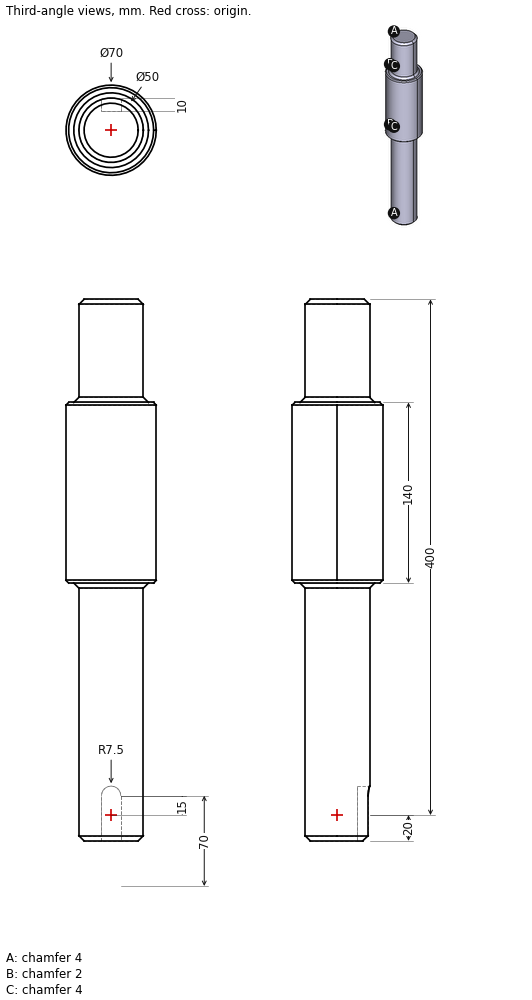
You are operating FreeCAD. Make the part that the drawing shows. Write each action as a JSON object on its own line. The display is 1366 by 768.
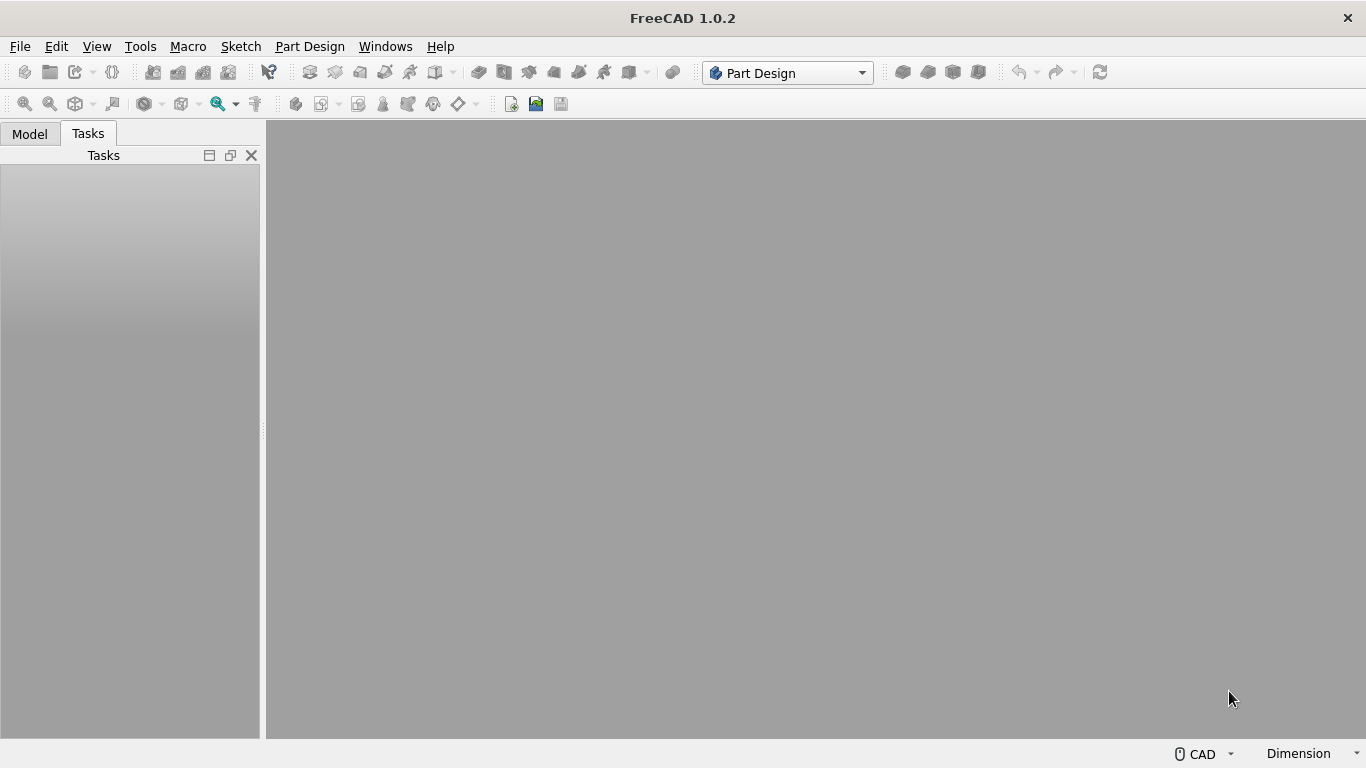
{"action": "left_click", "coordinate": [511, 104]}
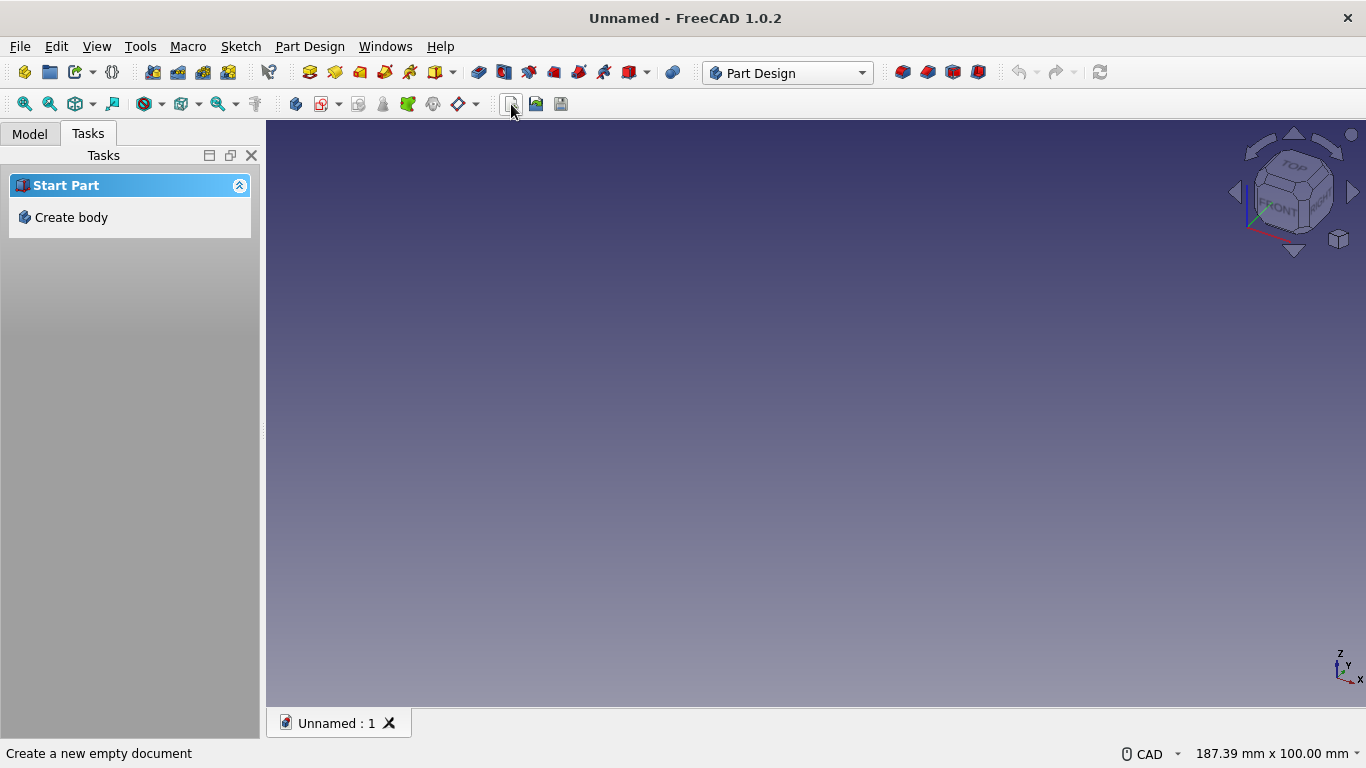
{"action": "left_click", "coordinate": [320, 104]}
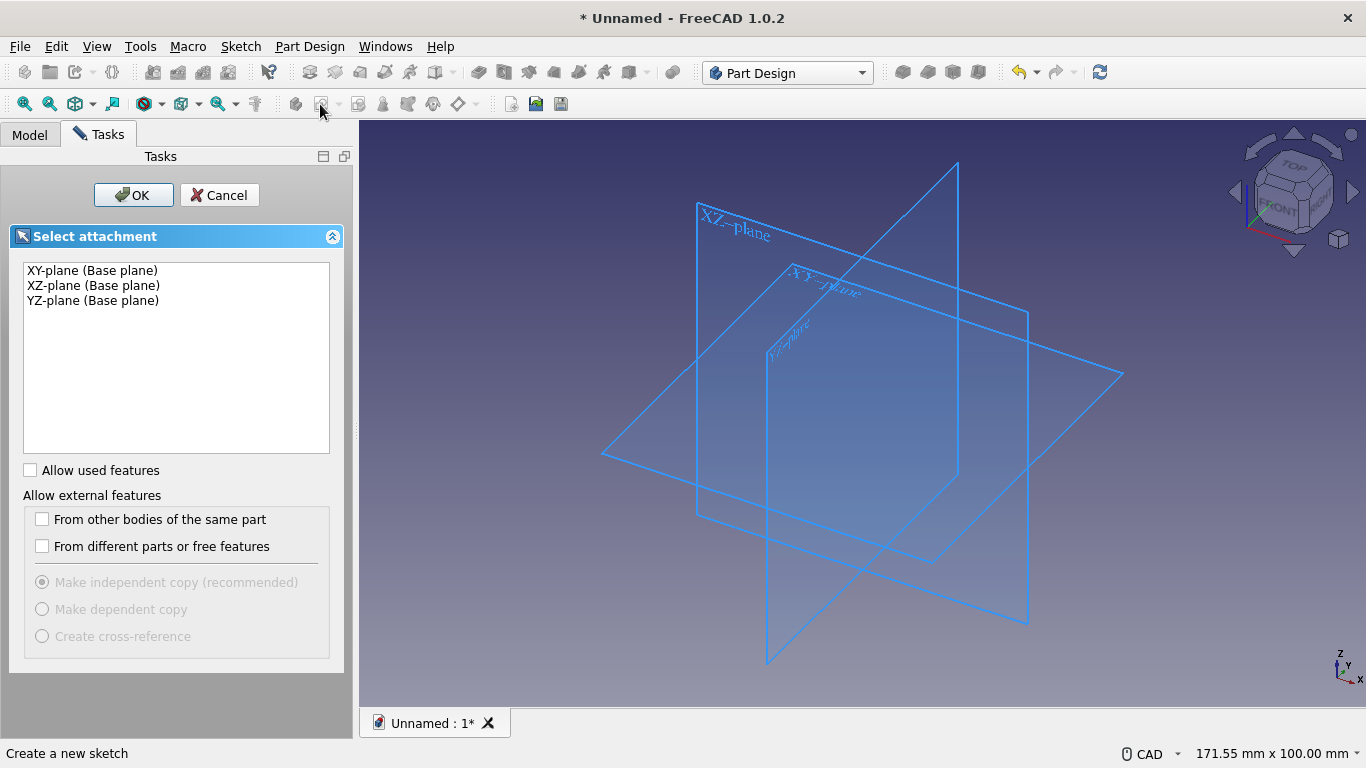
{"action": "left_click", "coordinate": [84, 270]}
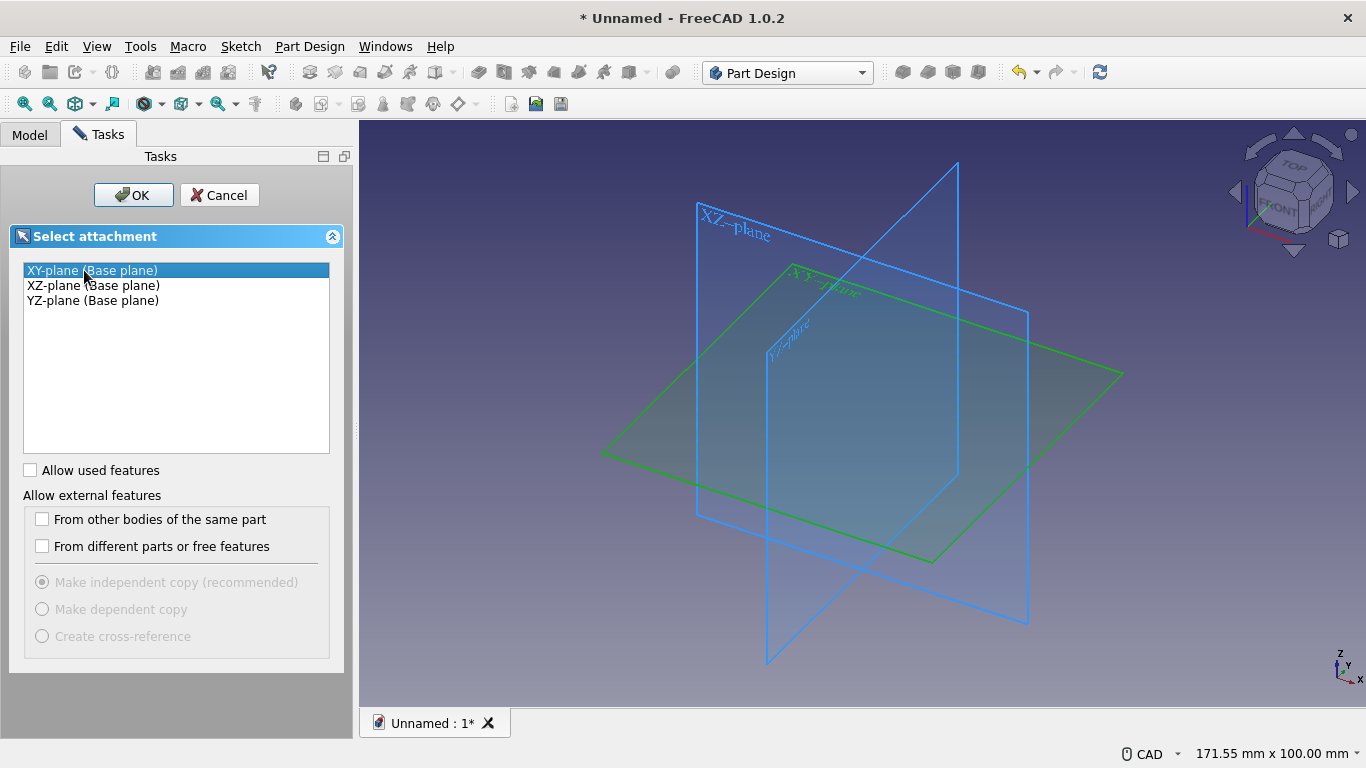
{"action": "left_click", "coordinate": [134, 195]}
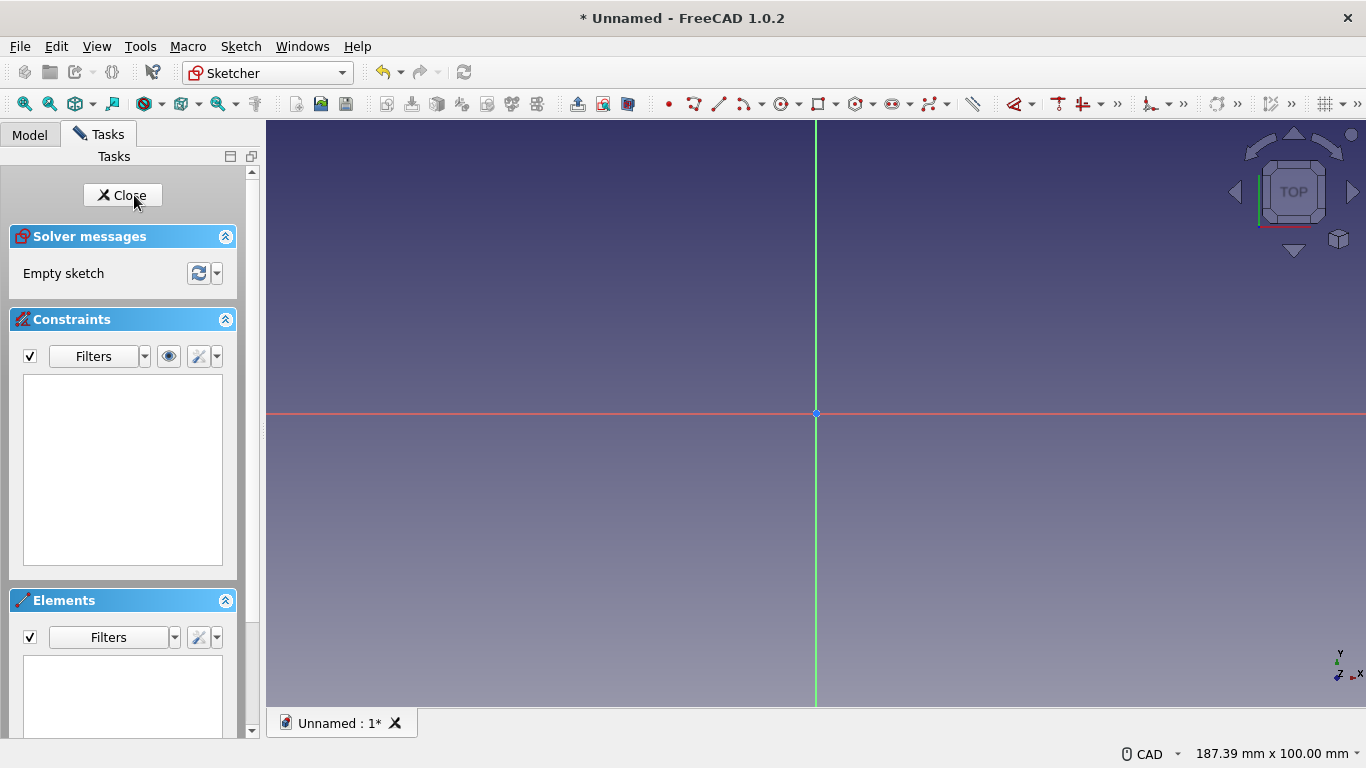
{"action": "left_click", "coordinate": [780, 104]}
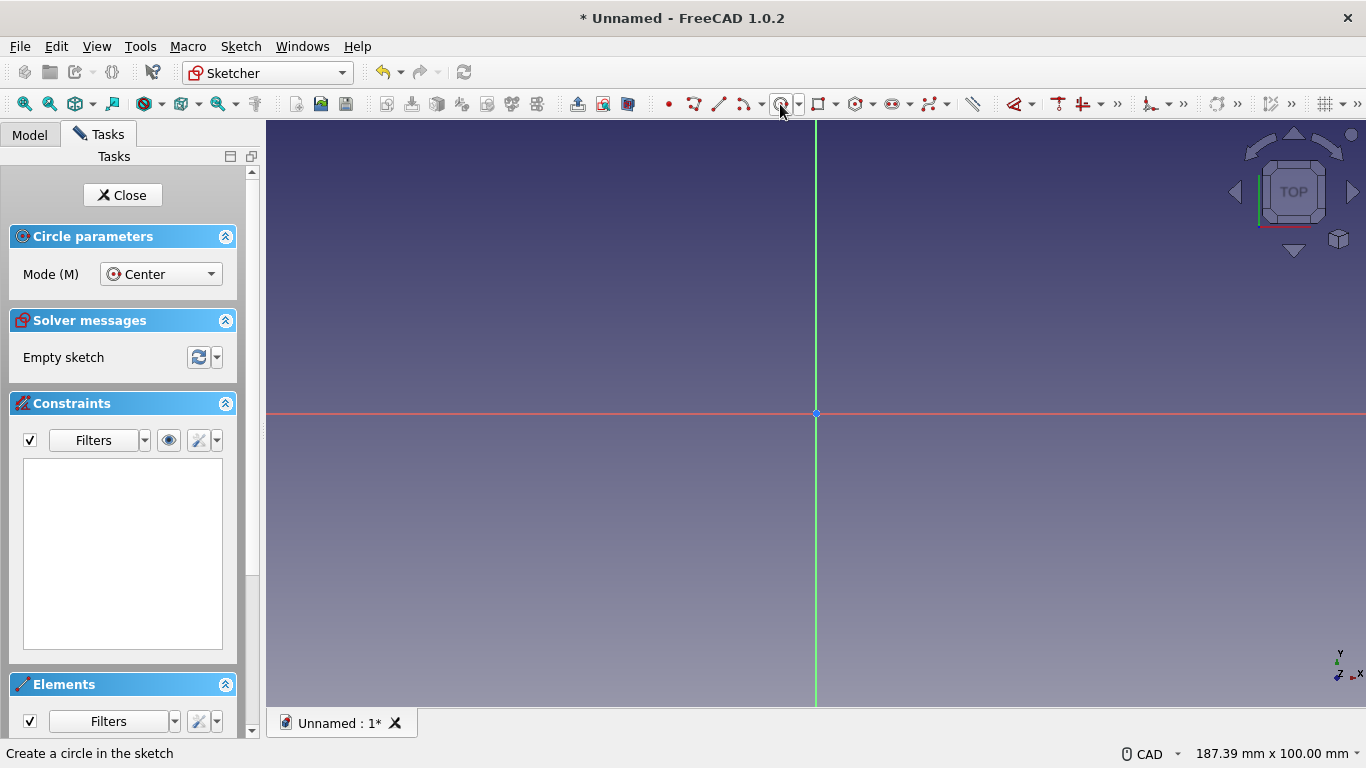
{"action": "left_click", "coordinate": [816, 414]}
{"action": "left_click", "coordinate": [920, 310]}
{"action": "key", "text": "Escape"}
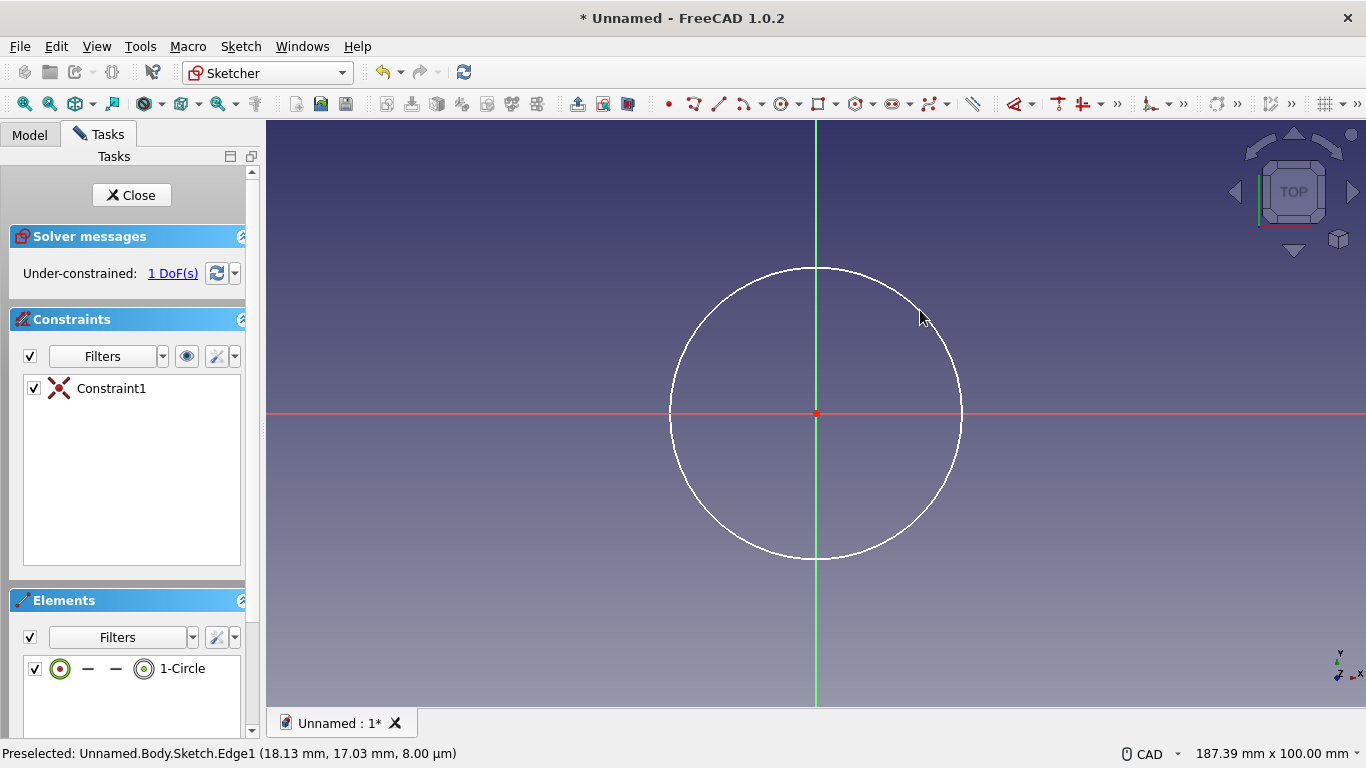
{"action": "left_click", "coordinate": [1014, 104]}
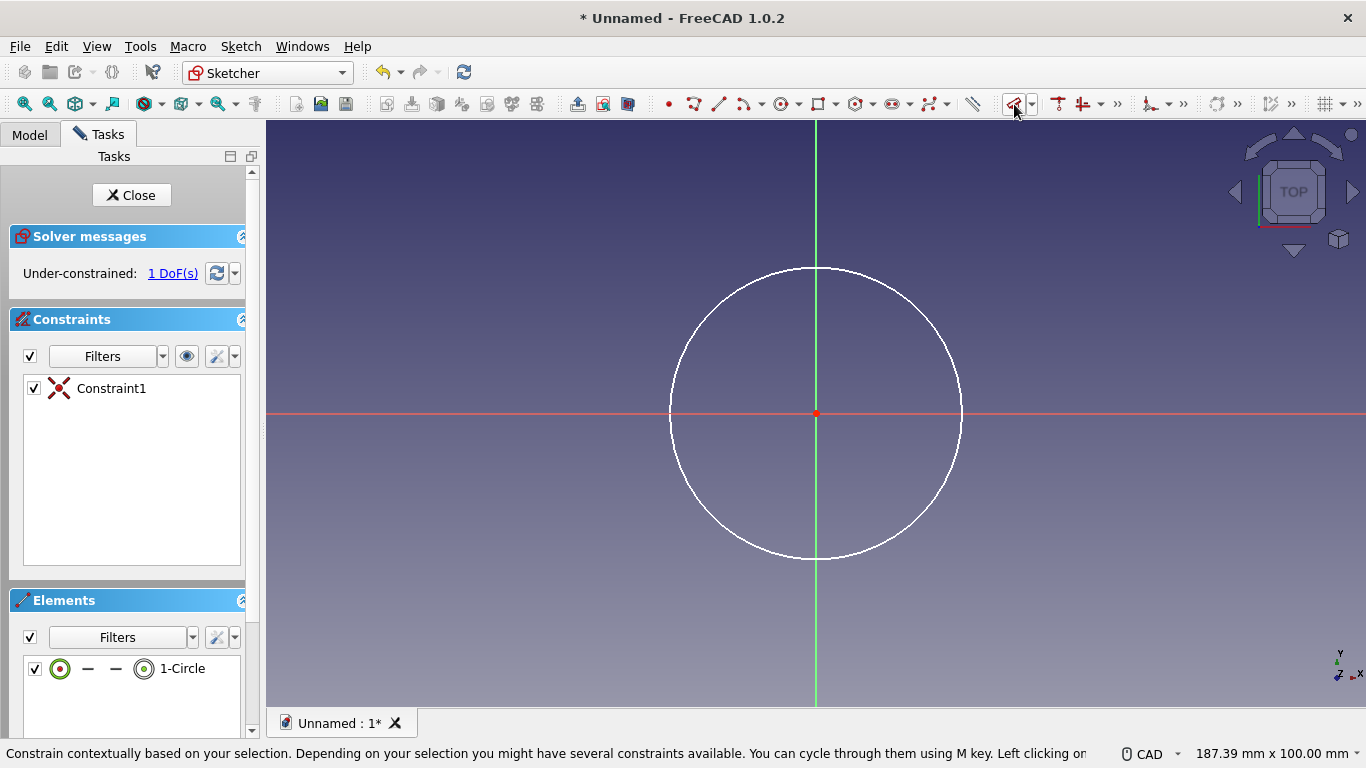
{"action": "left_click", "coordinate": [919, 310]}
{"action": "left_click", "coordinate": [942, 287]}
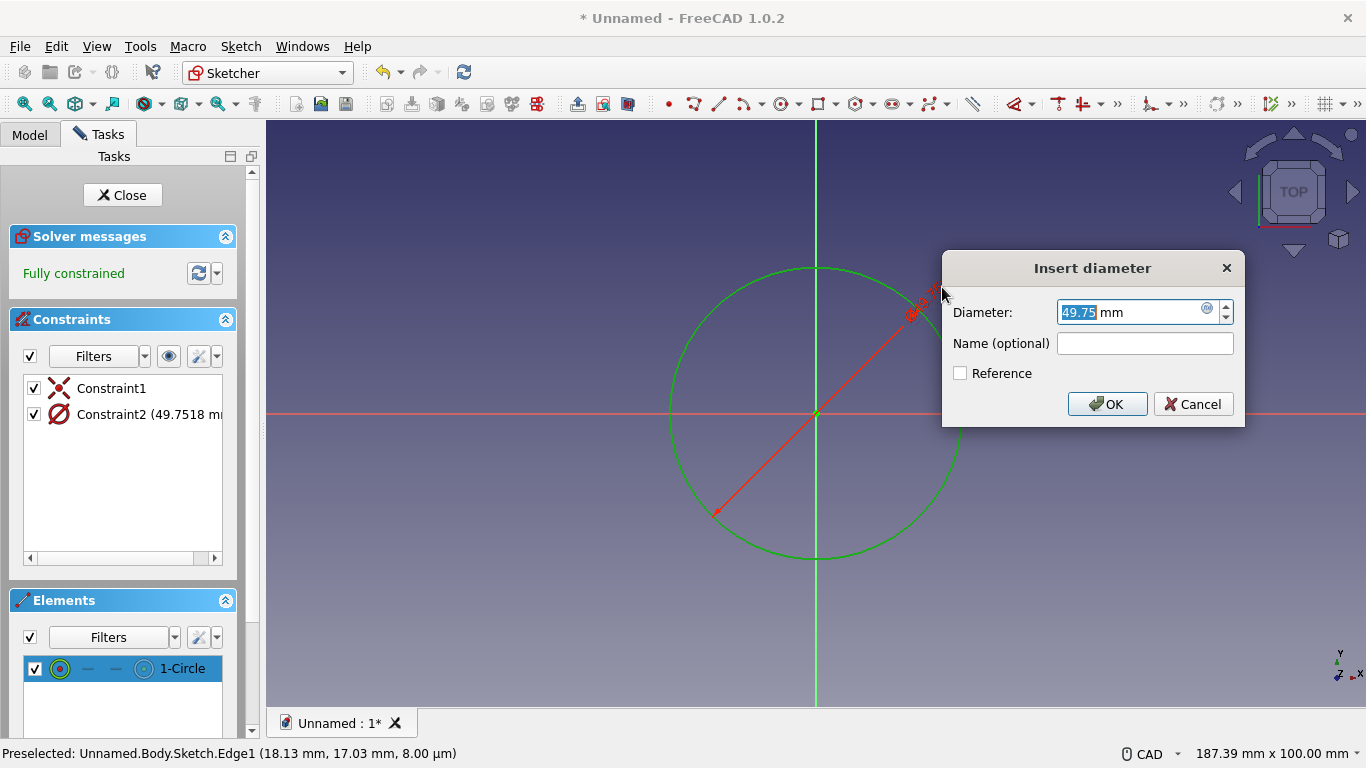
{"action": "type", "text": "50"}
{"action": "key", "text": "Return"}
{"action": "key", "text": "Escape"}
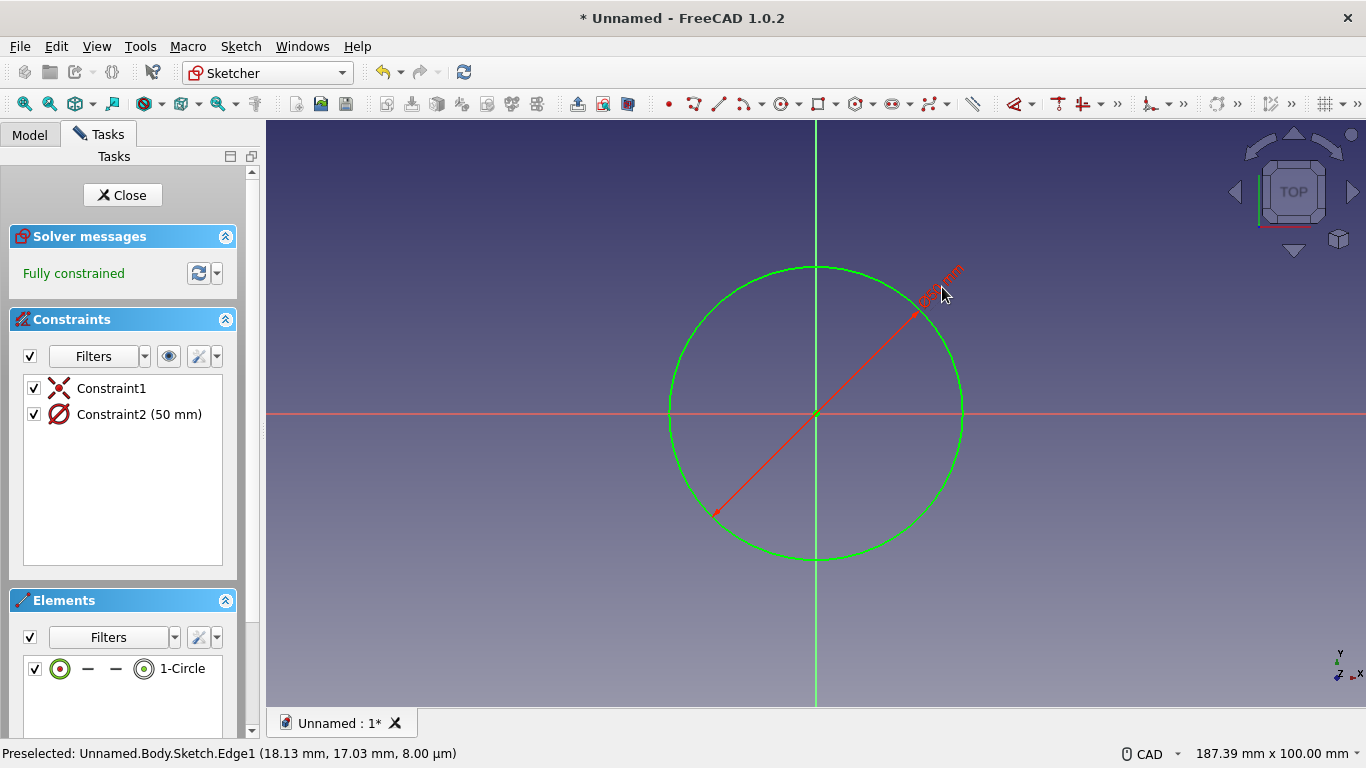
{"action": "left_click", "coordinate": [123, 195]}